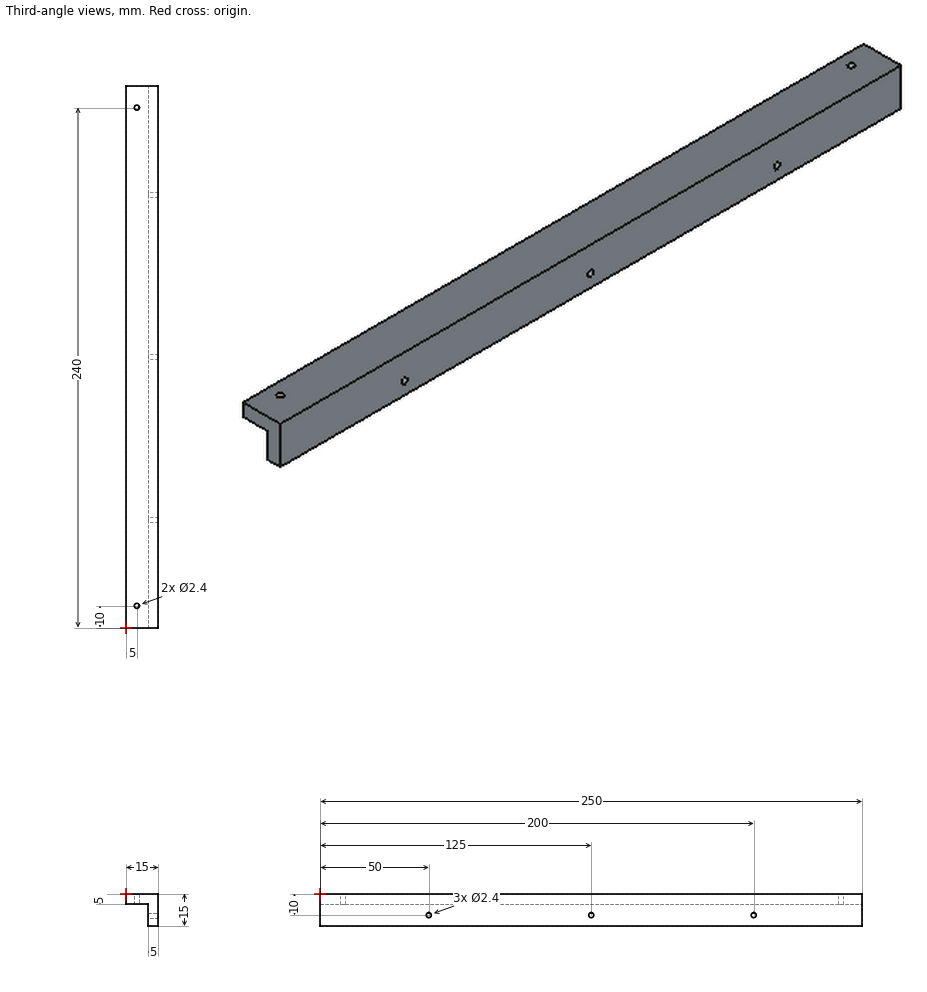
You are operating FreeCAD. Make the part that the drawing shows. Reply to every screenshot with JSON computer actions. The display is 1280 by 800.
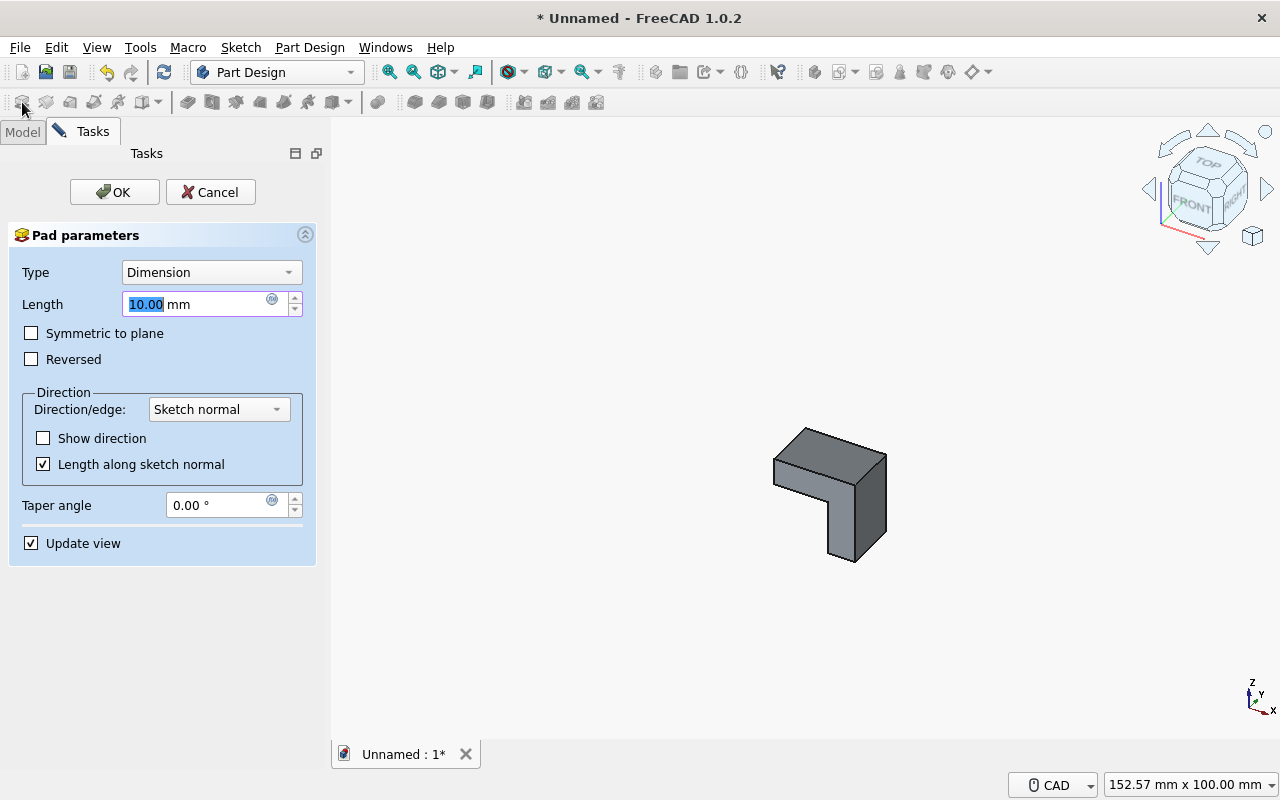
{"action": "type", "text": "250"}
{"action": "key", "text": "Tab"}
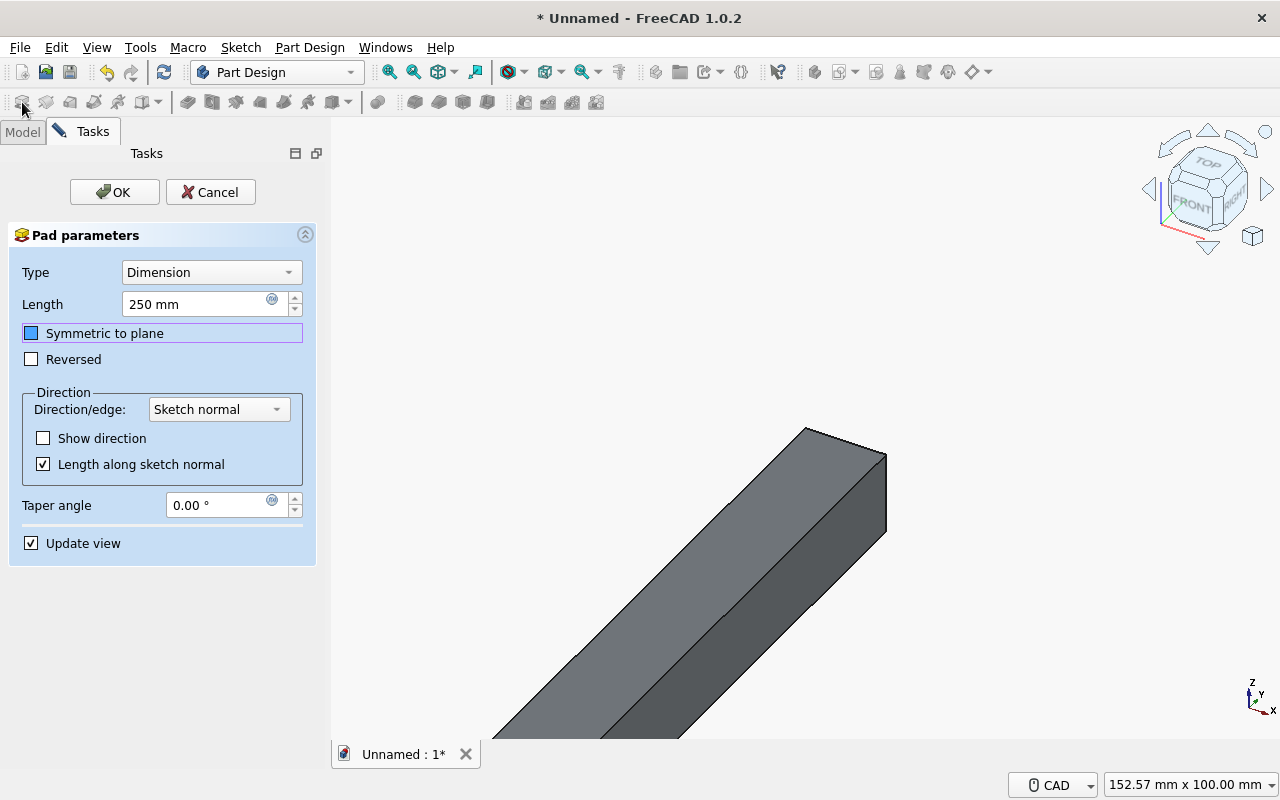
{"action": "left_click", "coordinate": [30, 359]}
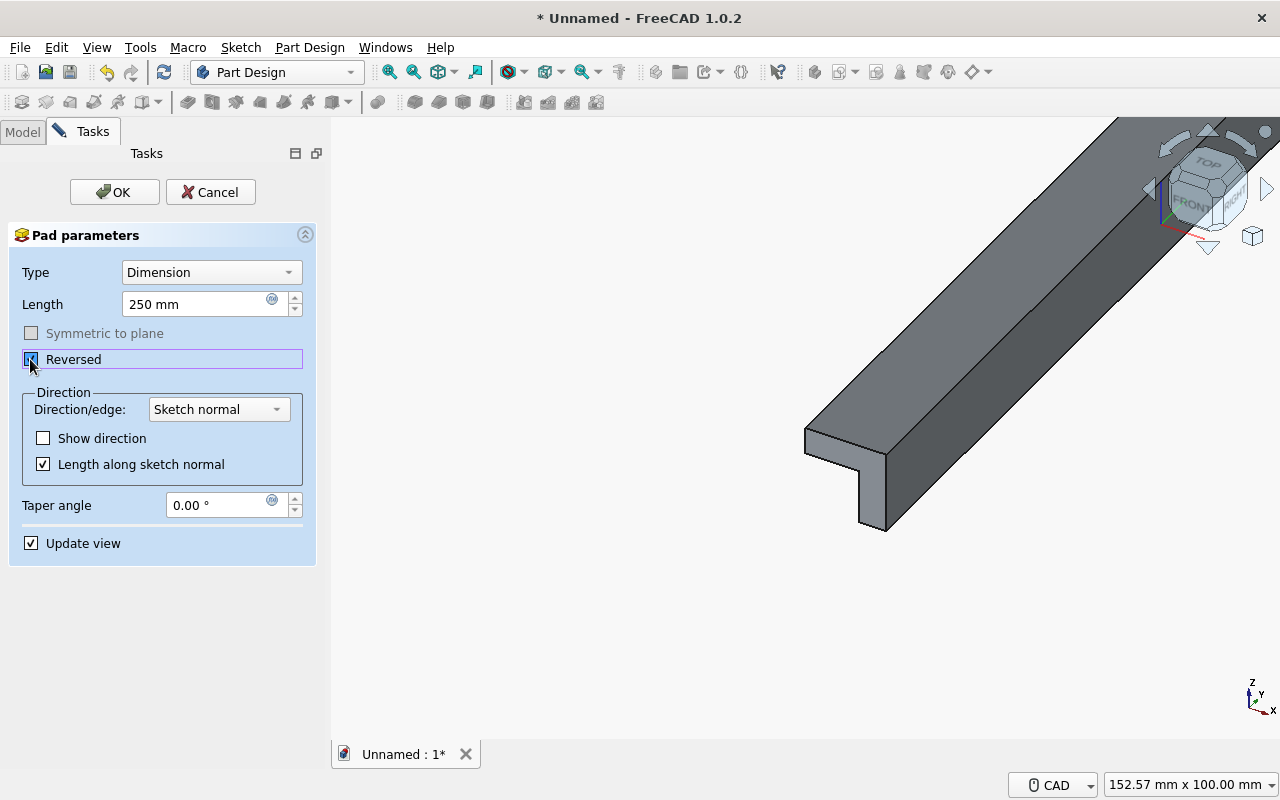
{"action": "left_click", "coordinate": [115, 192]}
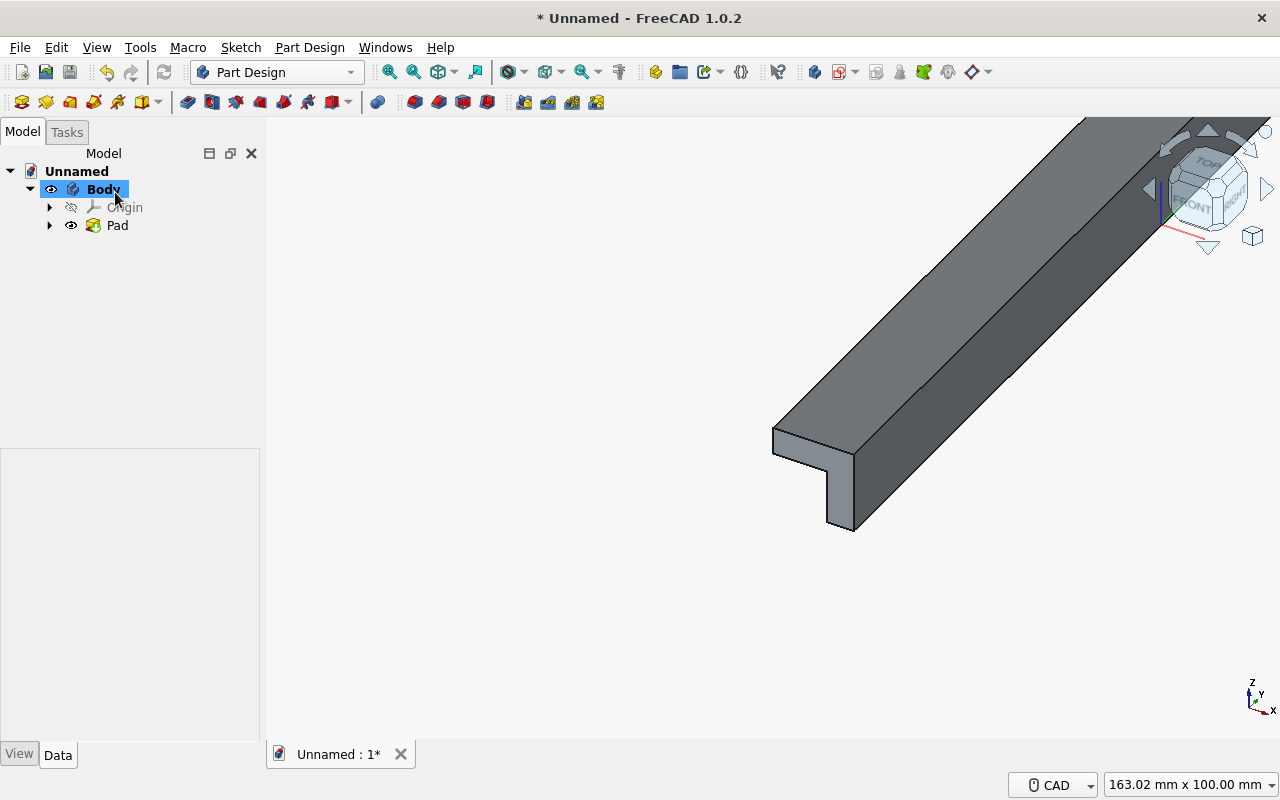
{"action": "key", "text": "v f"}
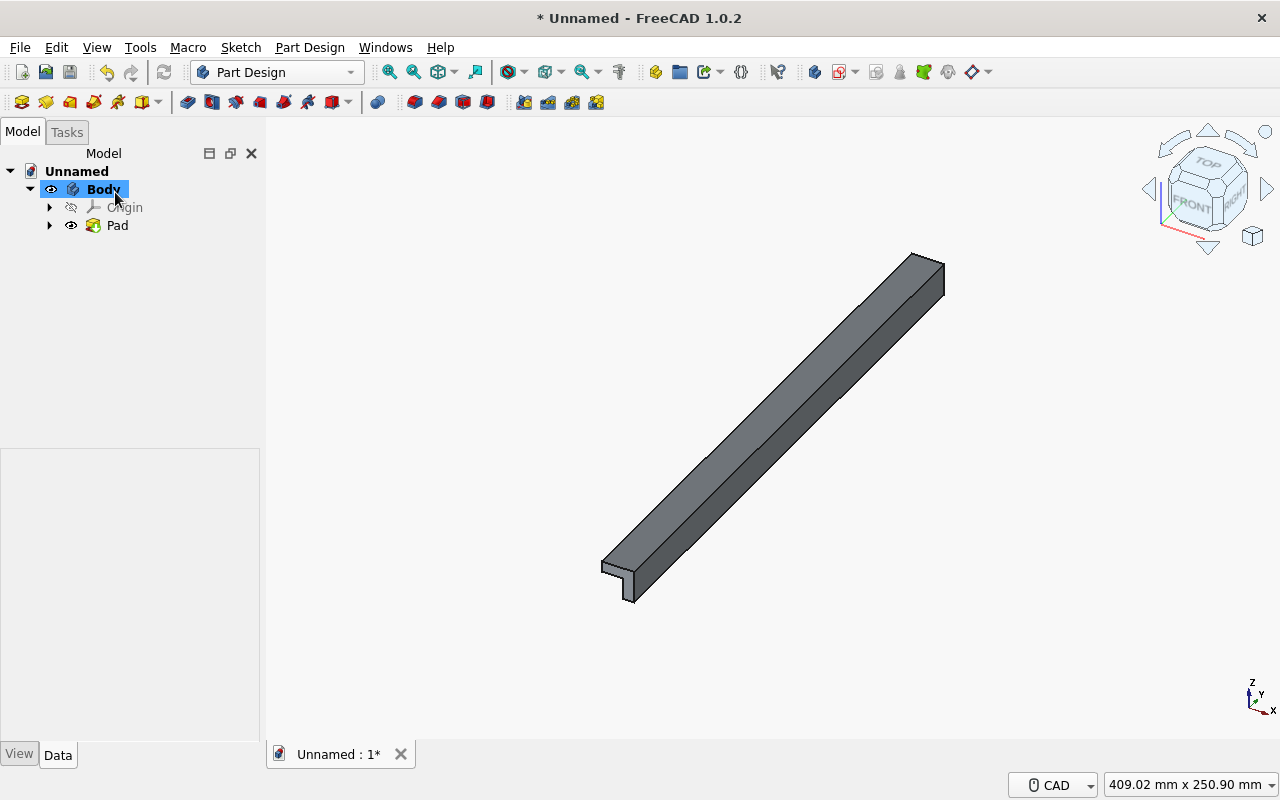
{"action": "key", "text": "6"}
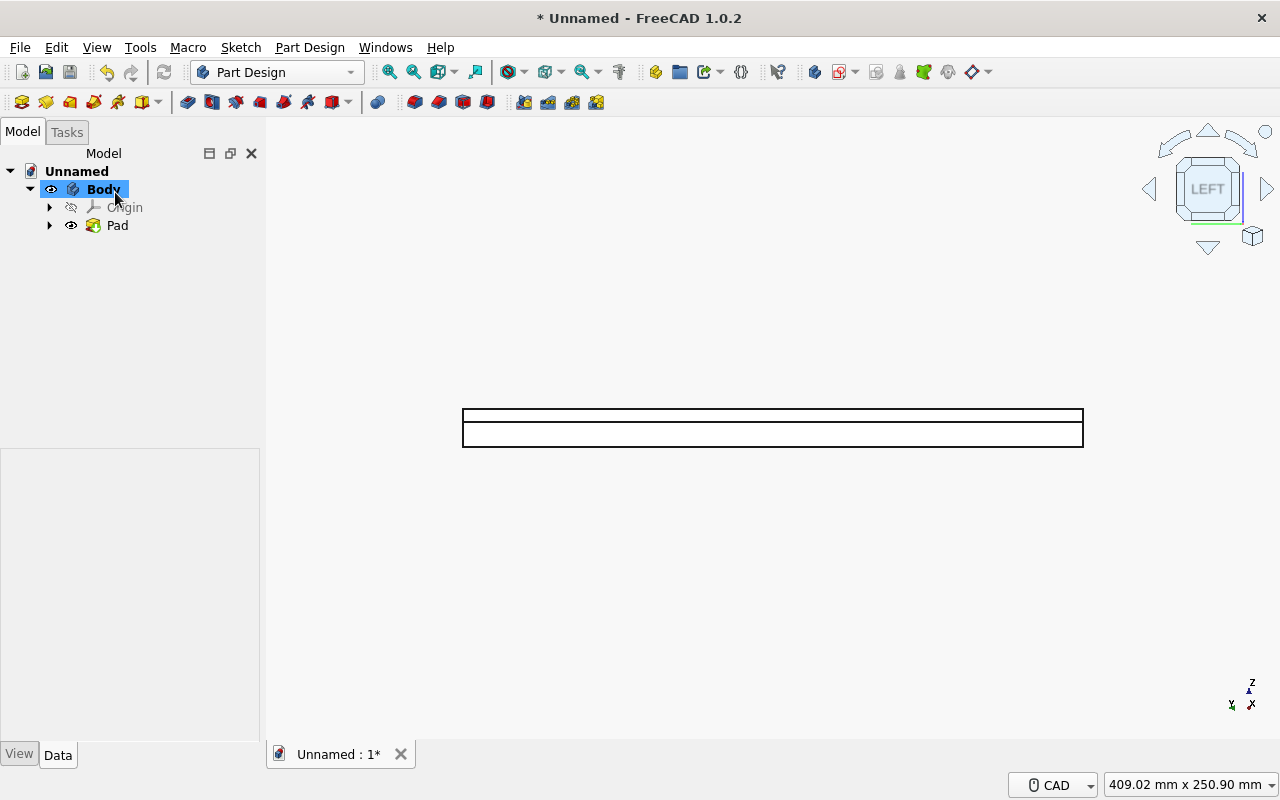
{"action": "left_click", "coordinate": [950, 433]}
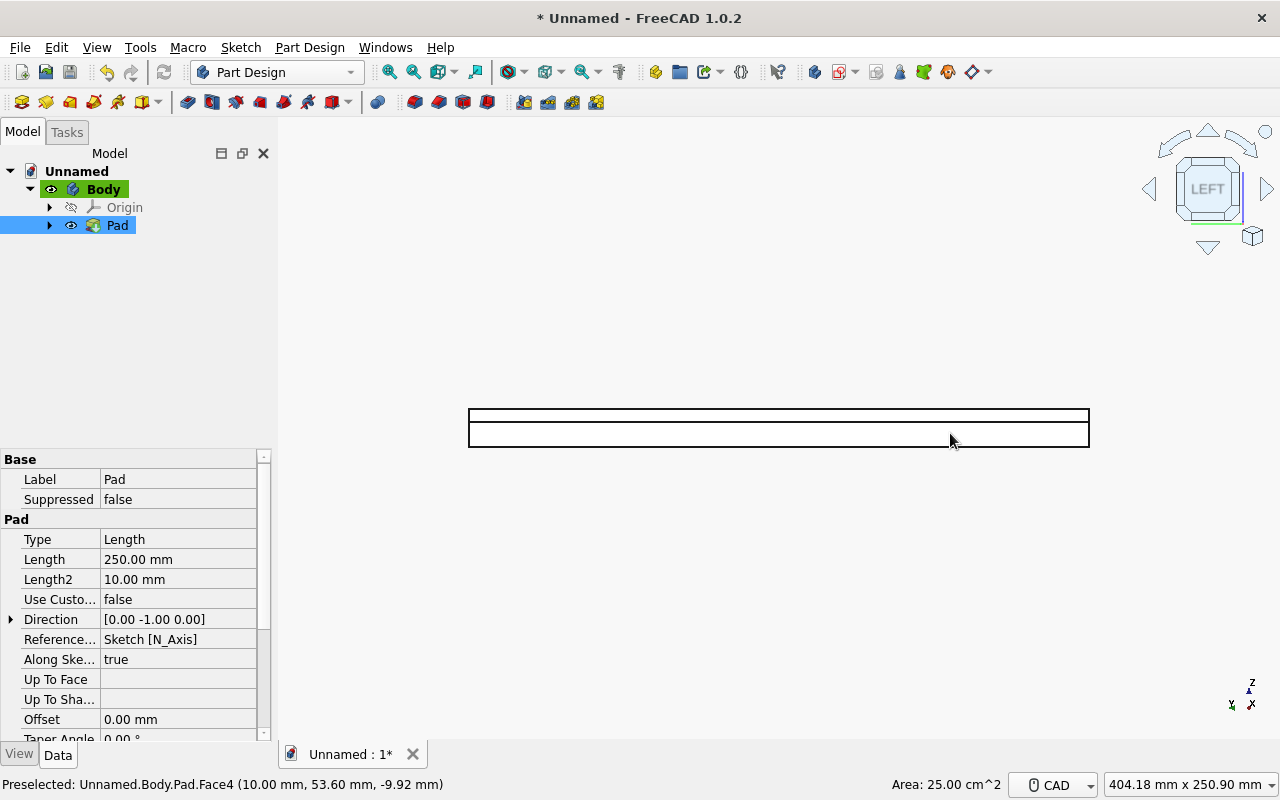
{"action": "left_click", "coordinate": [840, 72]}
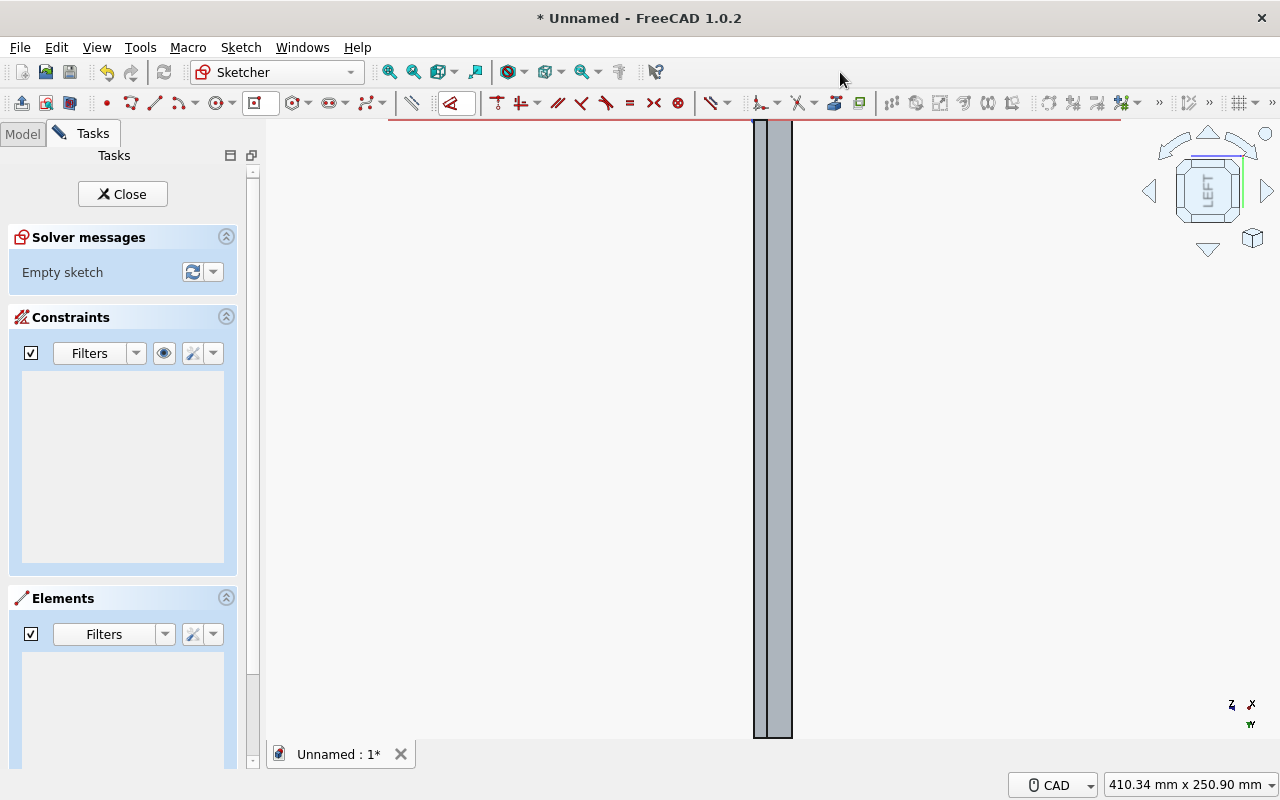
{"action": "scroll", "coordinate": [416, 701], "scroll_direction": "down", "scroll_amount": 1}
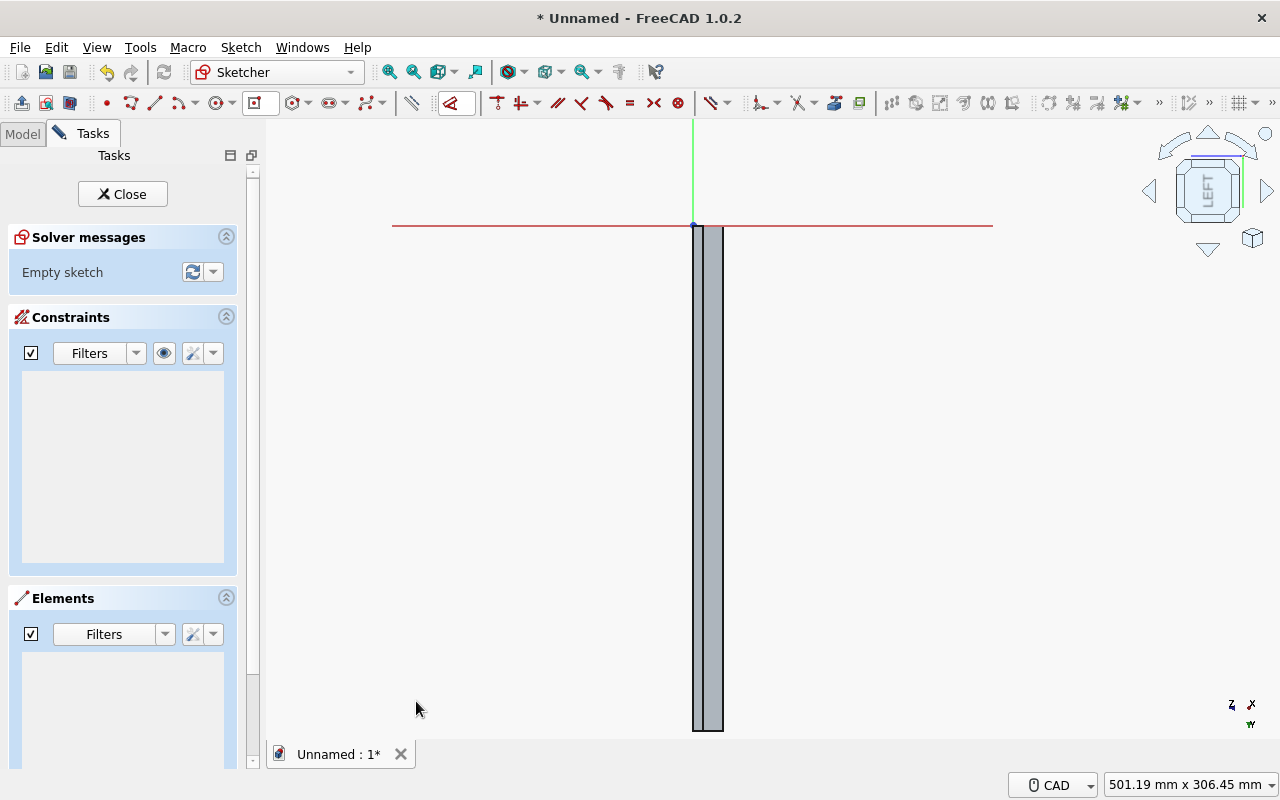
{"action": "left_click", "coordinate": [216, 104]}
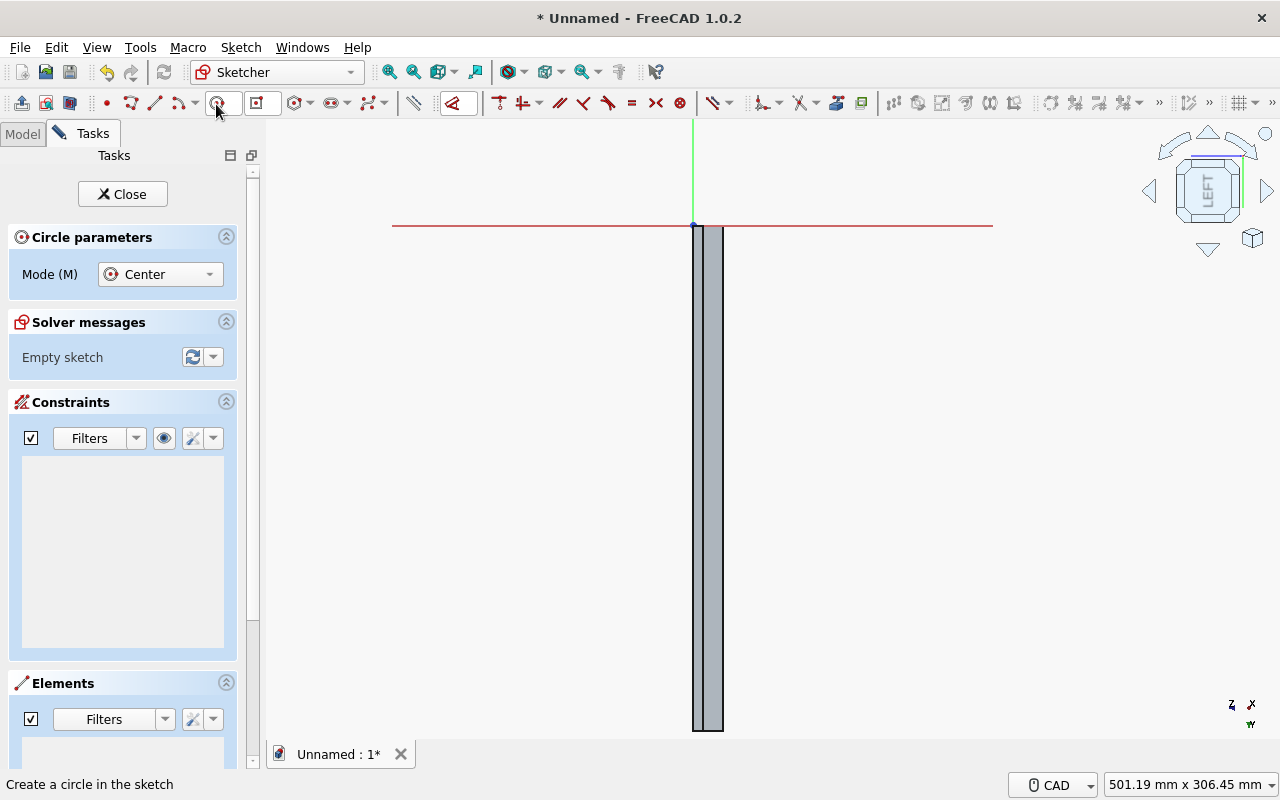
{"action": "scroll", "coordinate": [713, 327], "scroll_direction": "up", "scroll_amount": 12}